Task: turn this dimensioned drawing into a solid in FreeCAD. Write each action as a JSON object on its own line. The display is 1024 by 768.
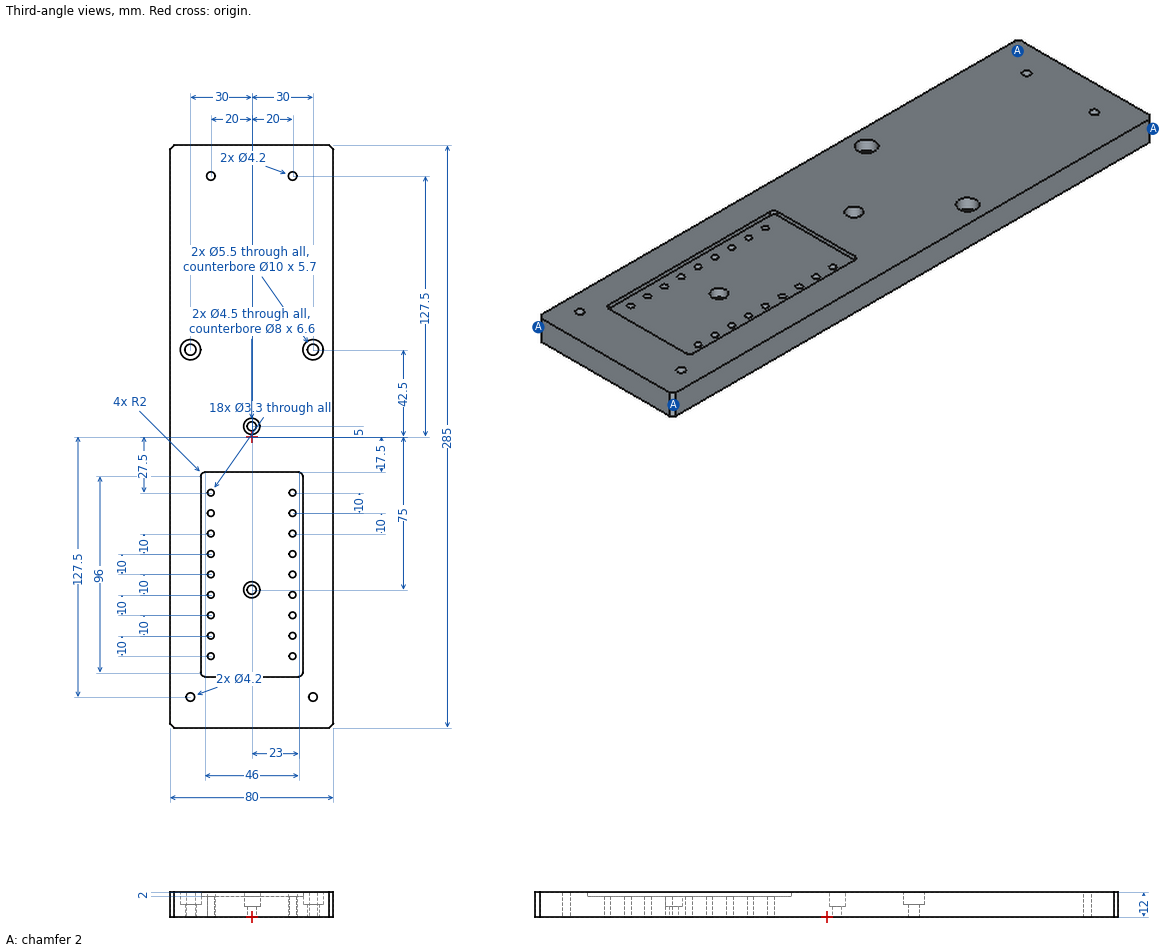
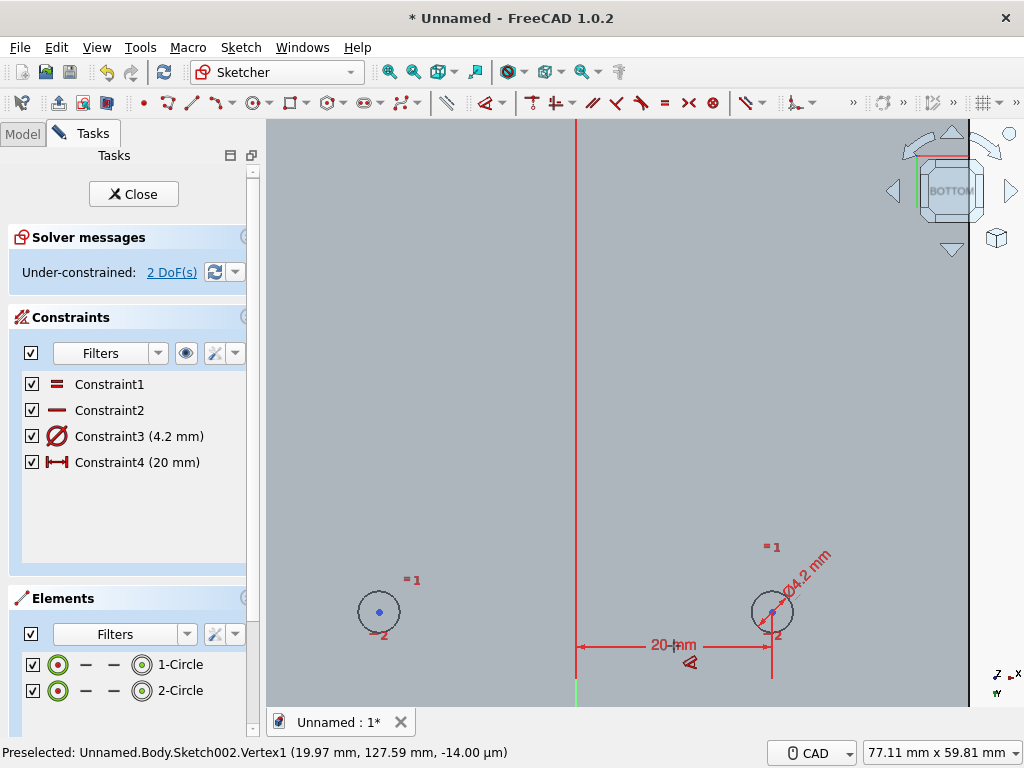
{"action": "left_click", "coordinate": [379, 612]}
{"action": "left_click", "coordinate": [477, 646]}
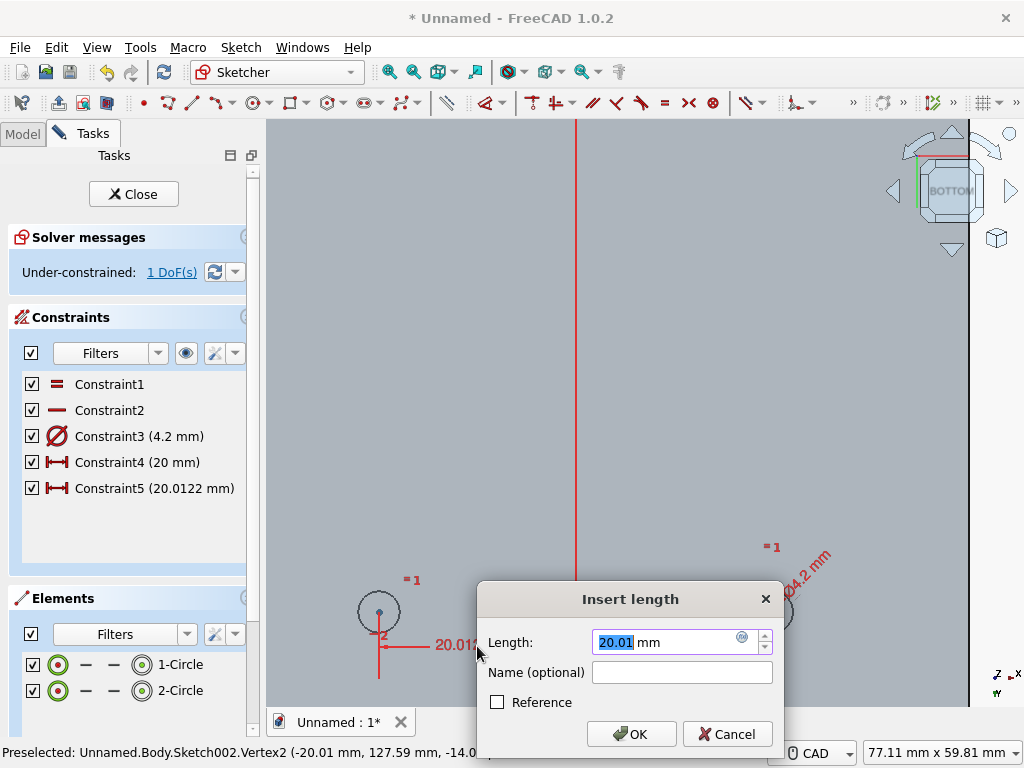
{"action": "type", "text": "20"}
{"action": "key", "text": "Return"}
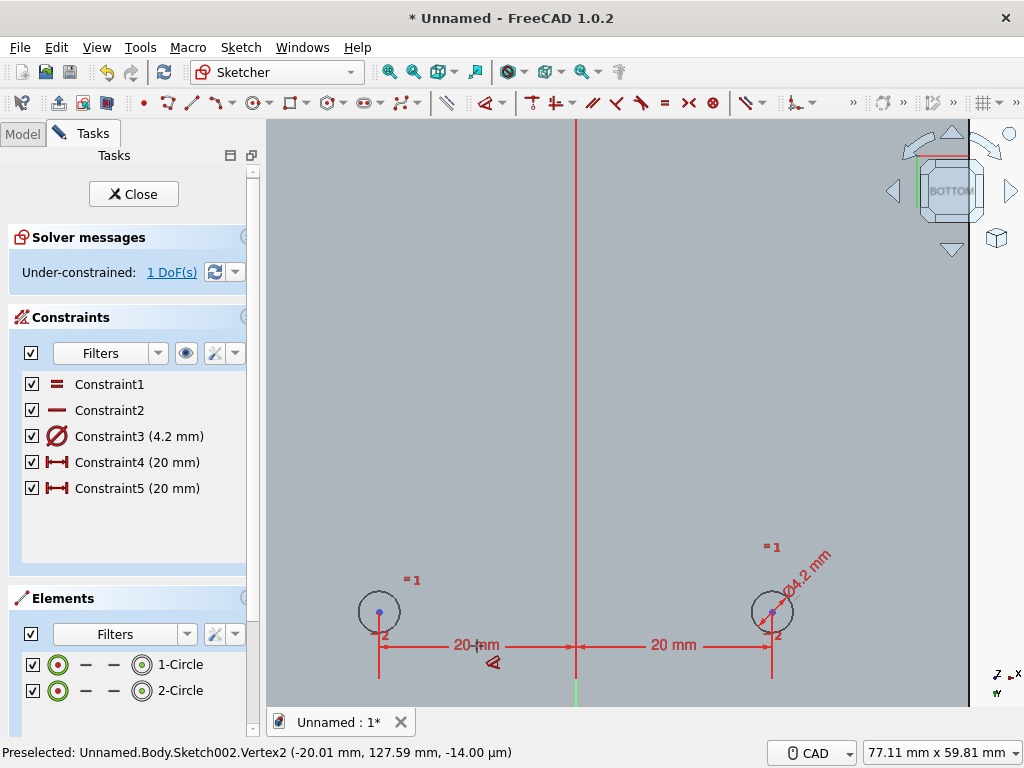
{"action": "left_click", "coordinate": [772, 612]}
{"action": "left_click", "coordinate": [806, 380]}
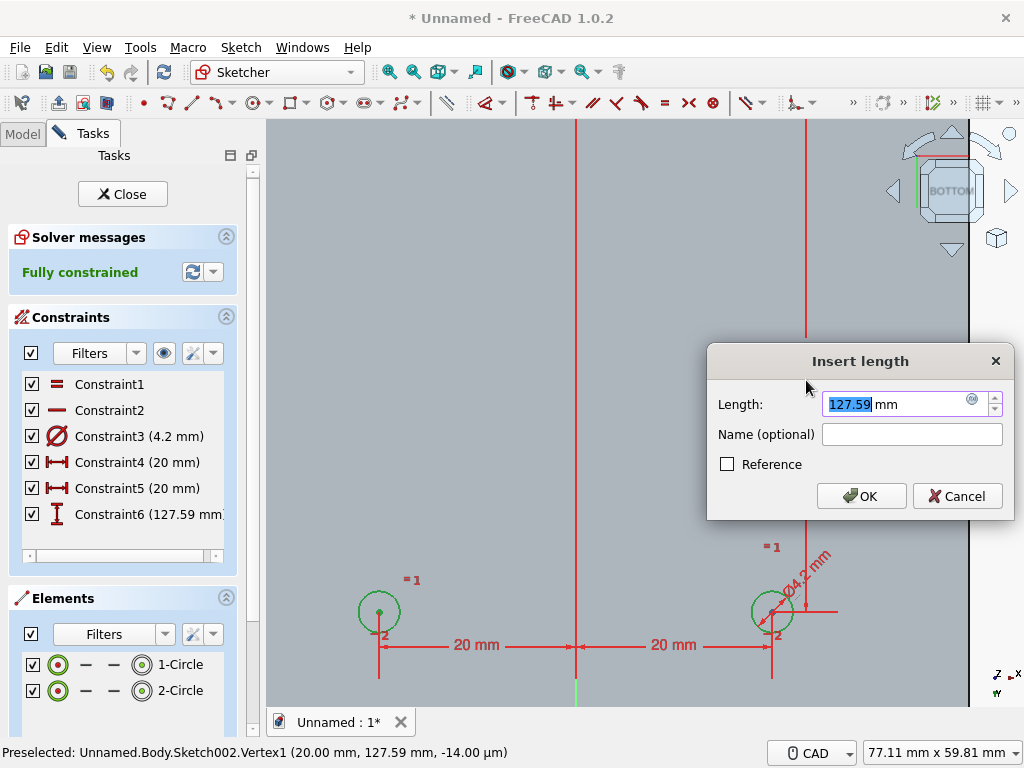
{"action": "type", "text": "127.5"}
{"action": "key", "text": "Return"}
{"action": "key", "text": "Escape"}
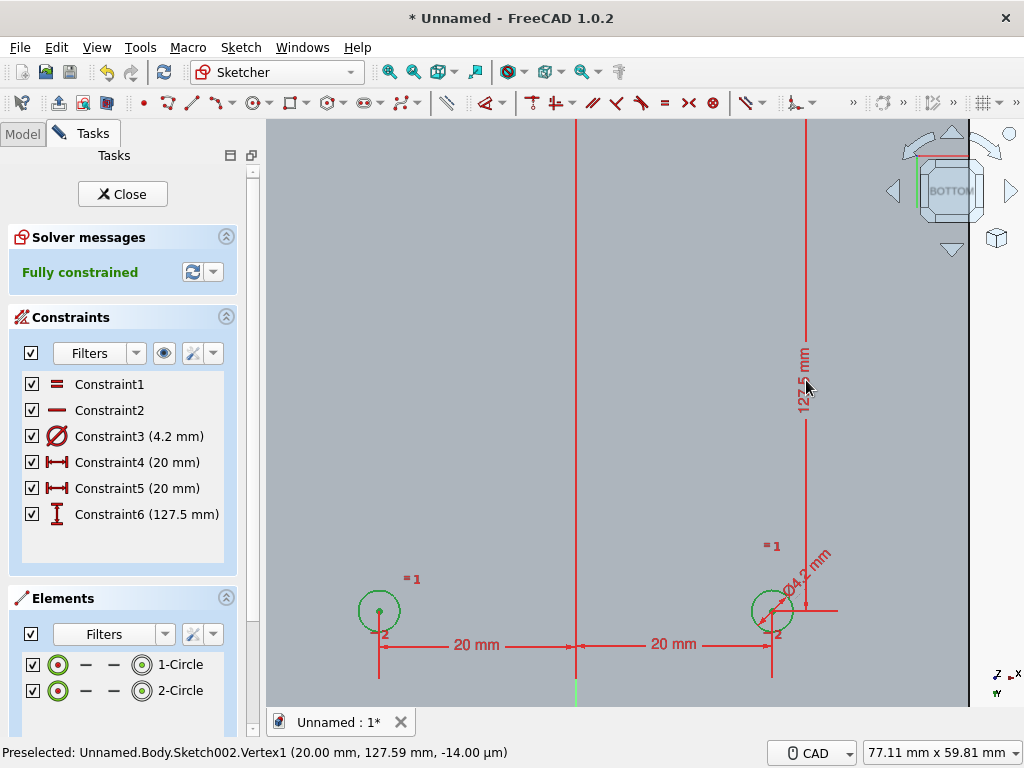
{"action": "left_click", "coordinate": [123, 194]}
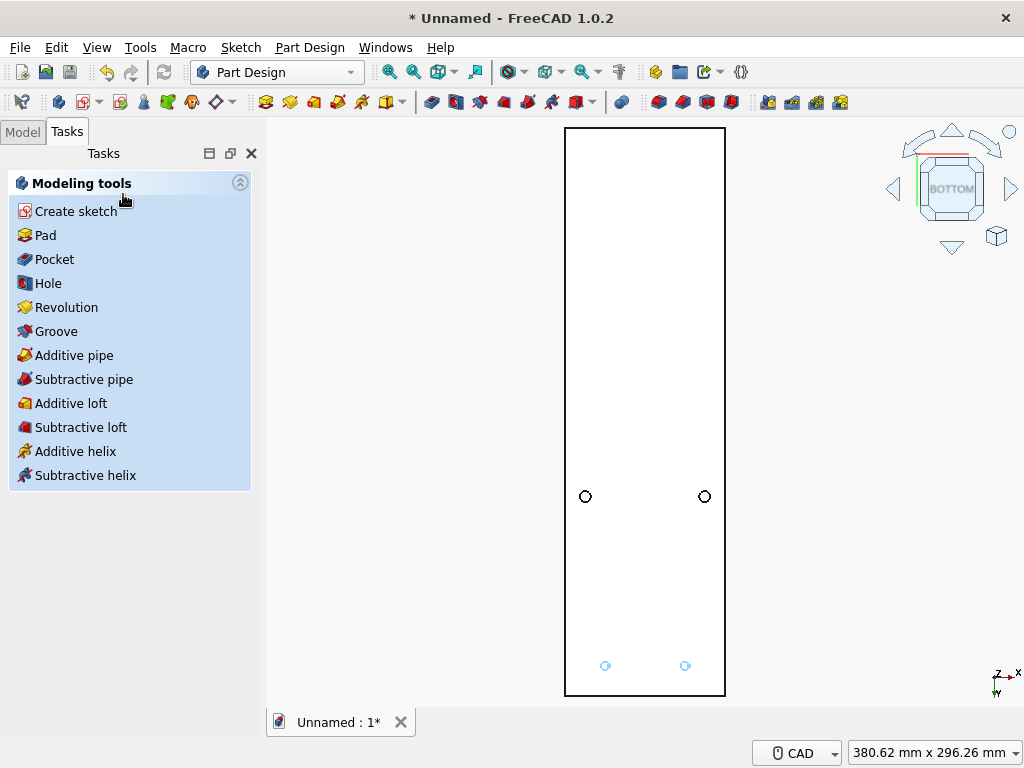
{"action": "left_click", "coordinate": [432, 102]}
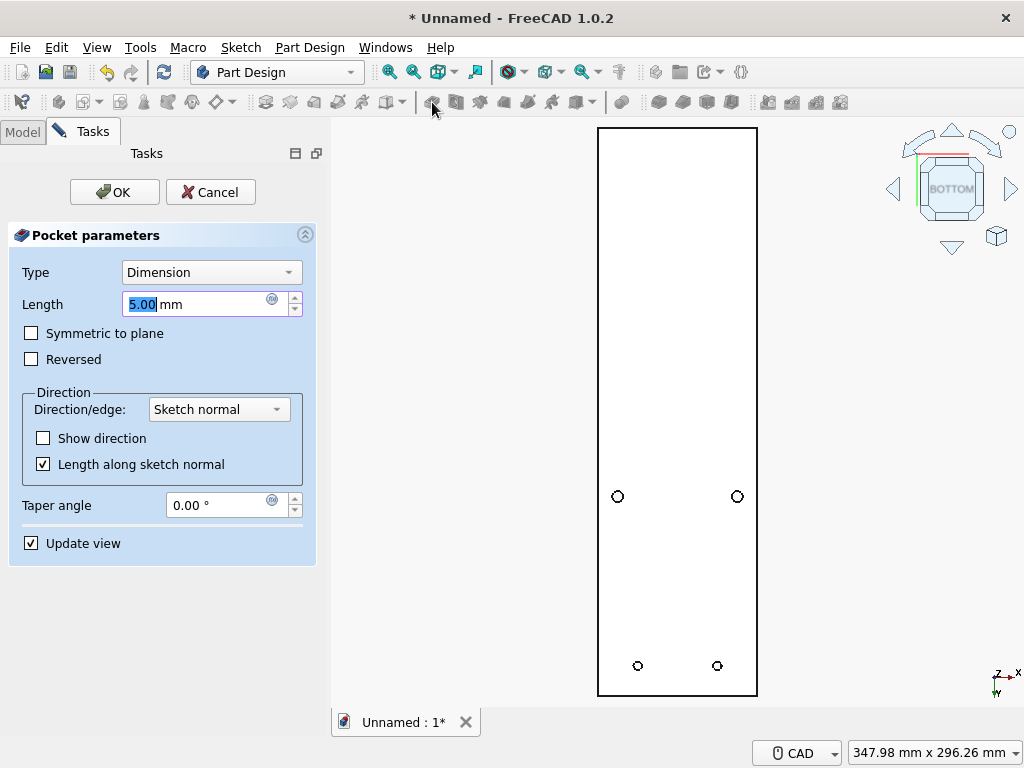
{"action": "left_click", "coordinate": [212, 272]}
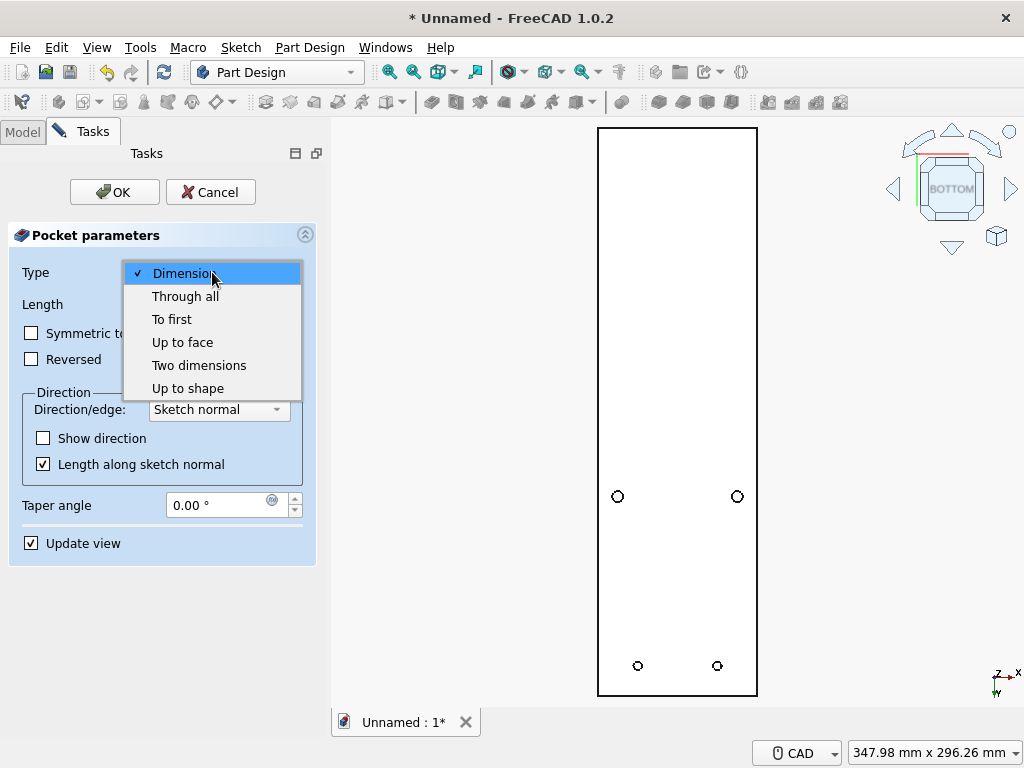
{"action": "left_click", "coordinate": [212, 296]}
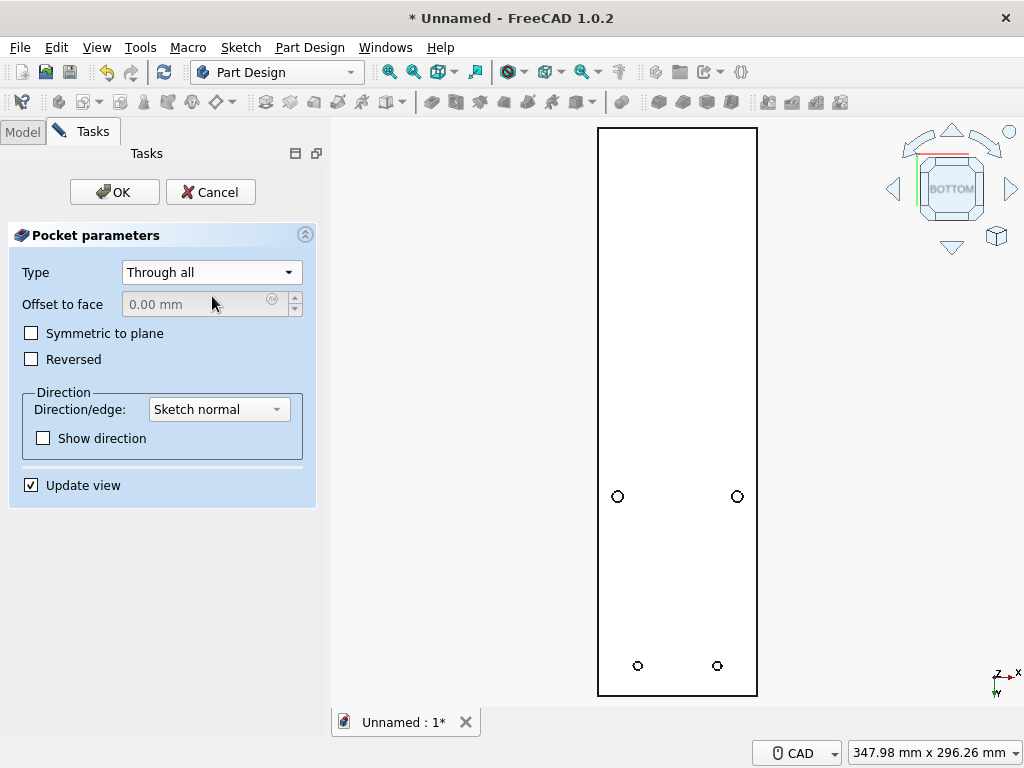
{"action": "left_click", "coordinate": [115, 192]}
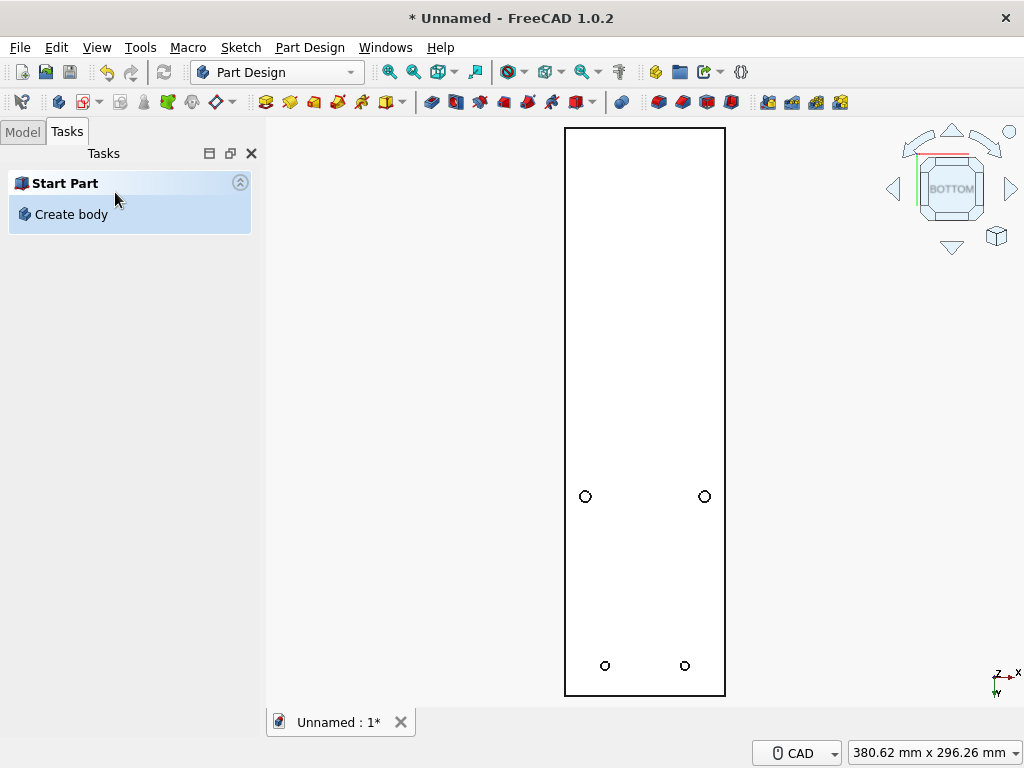
{"action": "key", "text": "0"}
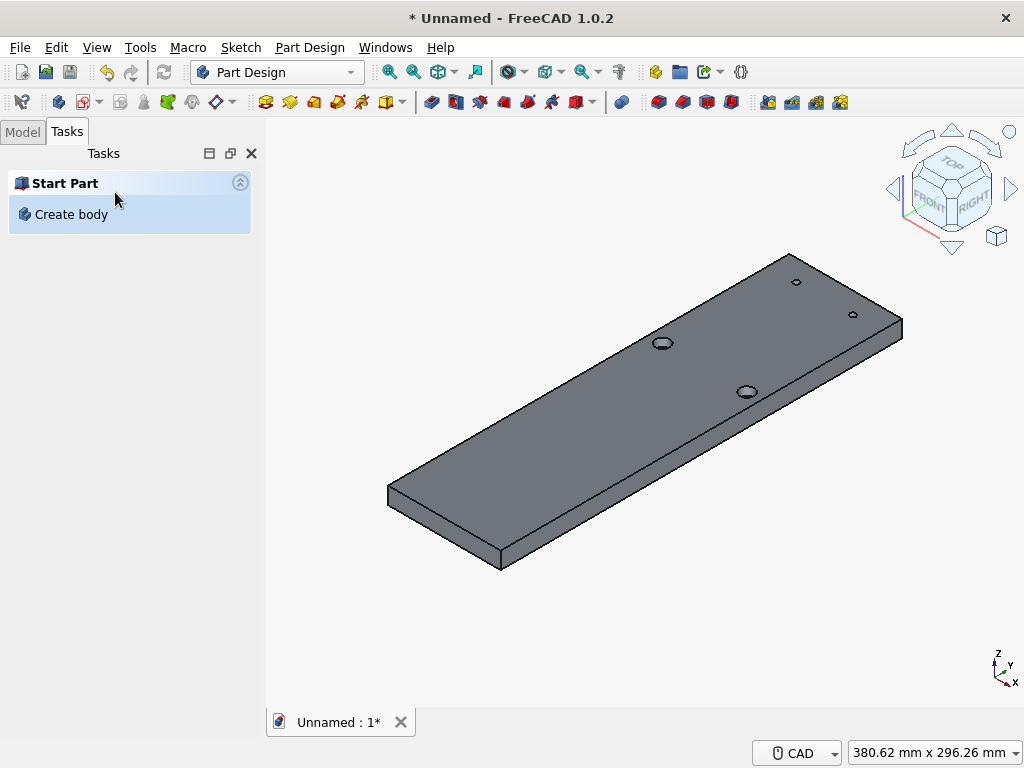
{"action": "left_click", "coordinate": [760, 335]}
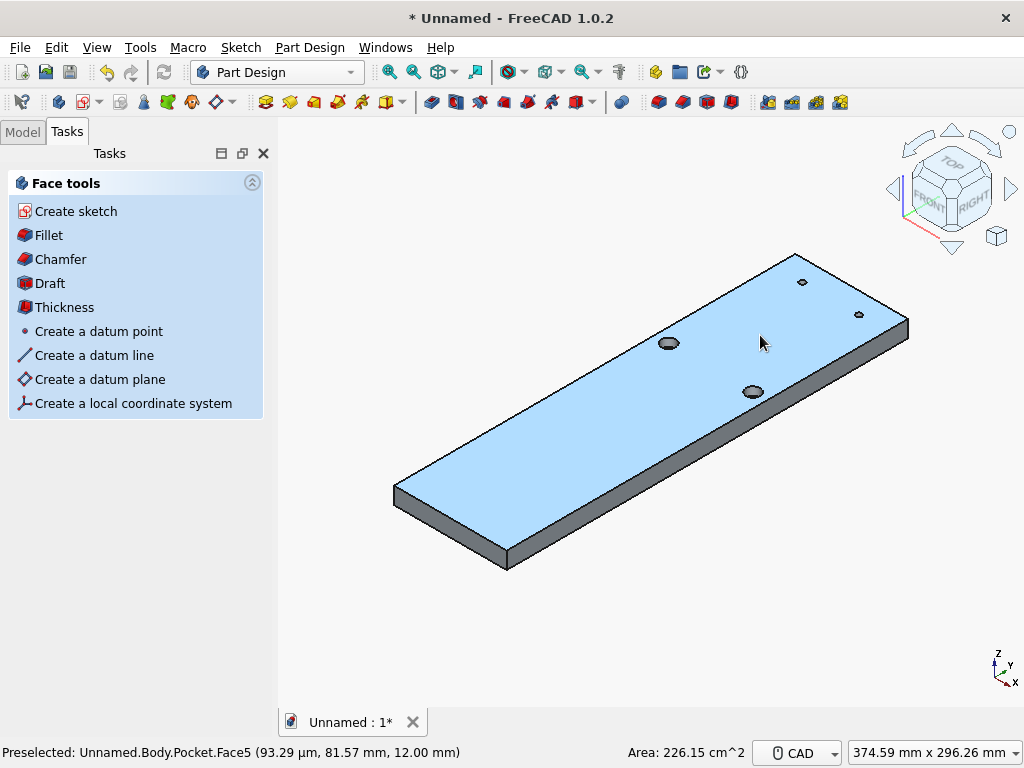
{"action": "left_click", "coordinate": [84, 102]}